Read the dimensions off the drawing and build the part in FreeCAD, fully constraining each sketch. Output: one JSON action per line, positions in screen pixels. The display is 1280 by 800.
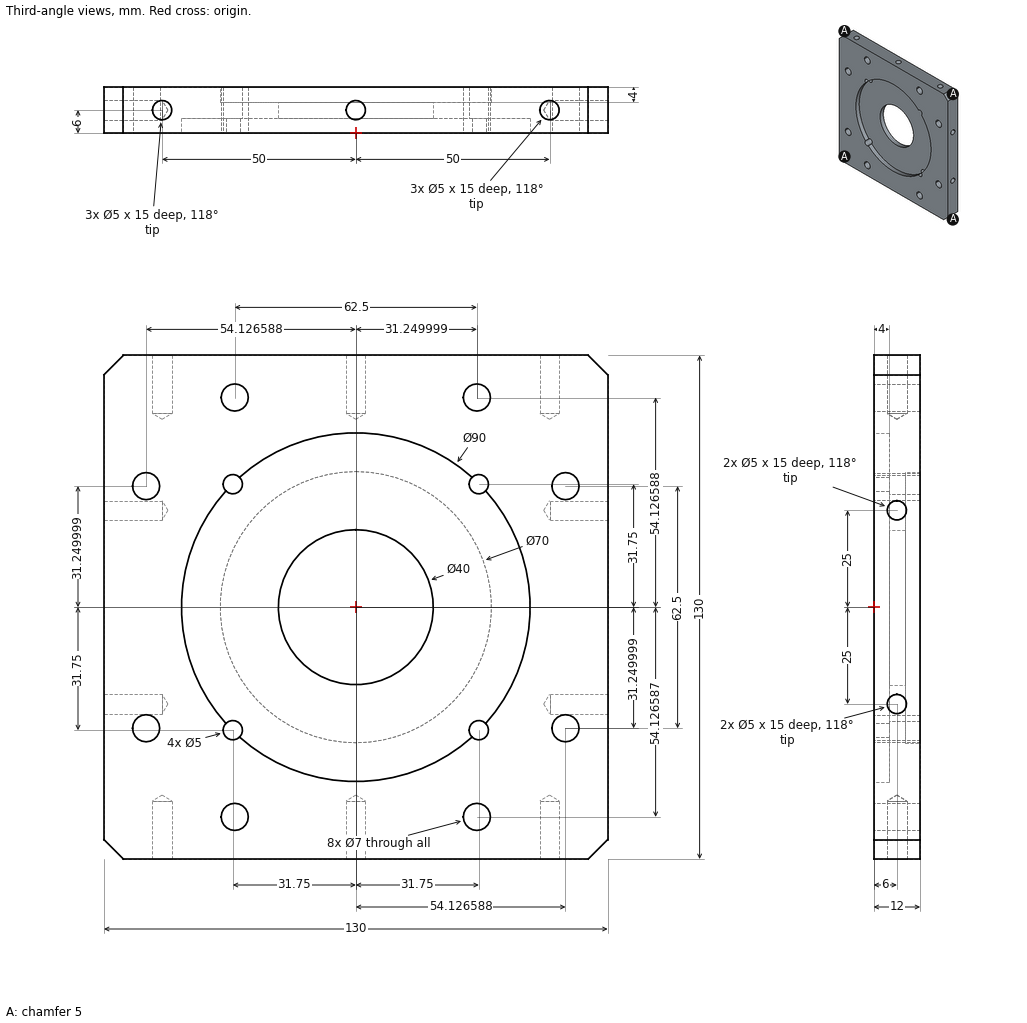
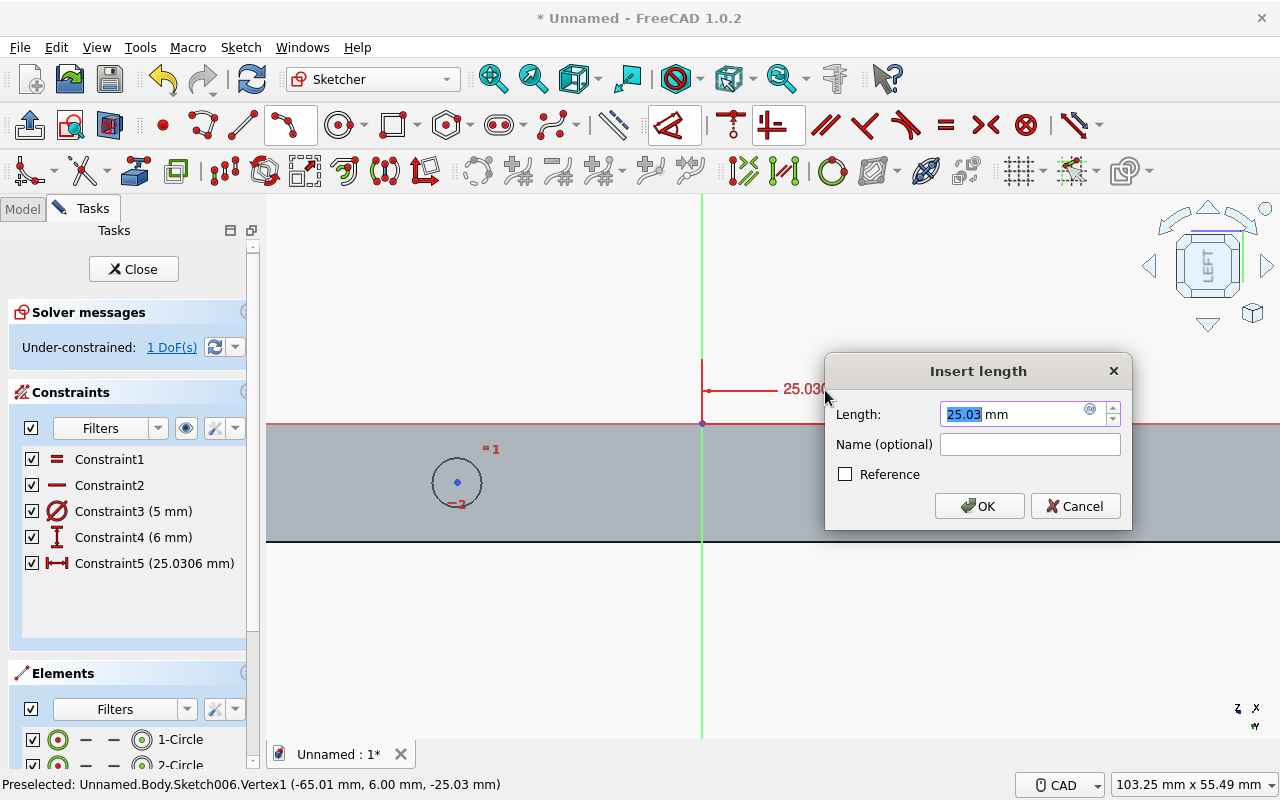
{"action": "type", "text": "25"}
{"action": "key", "text": "Return"}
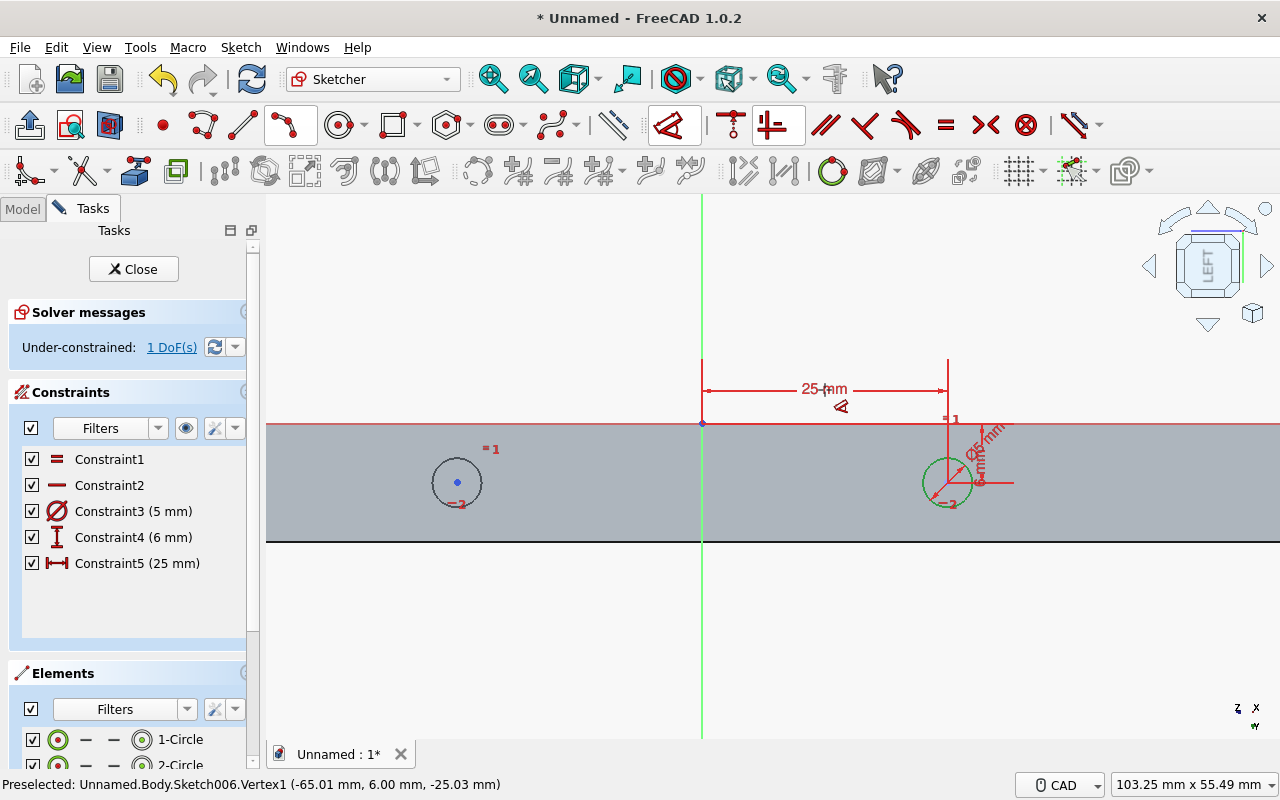
{"action": "left_click", "coordinate": [457, 483]}
{"action": "left_click", "coordinate": [580, 390]}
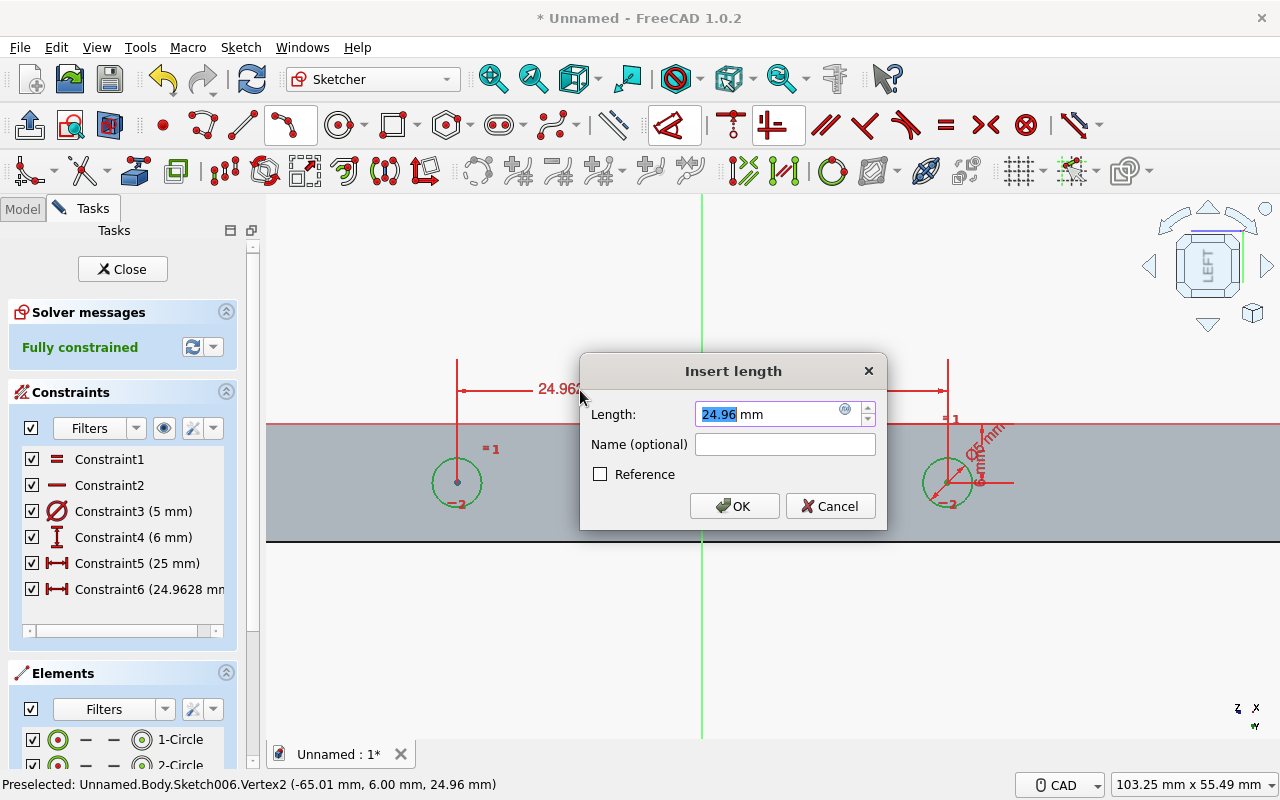
{"action": "type", "text": "25"}
{"action": "key", "text": "Return"}
{"action": "key", "text": "Escape"}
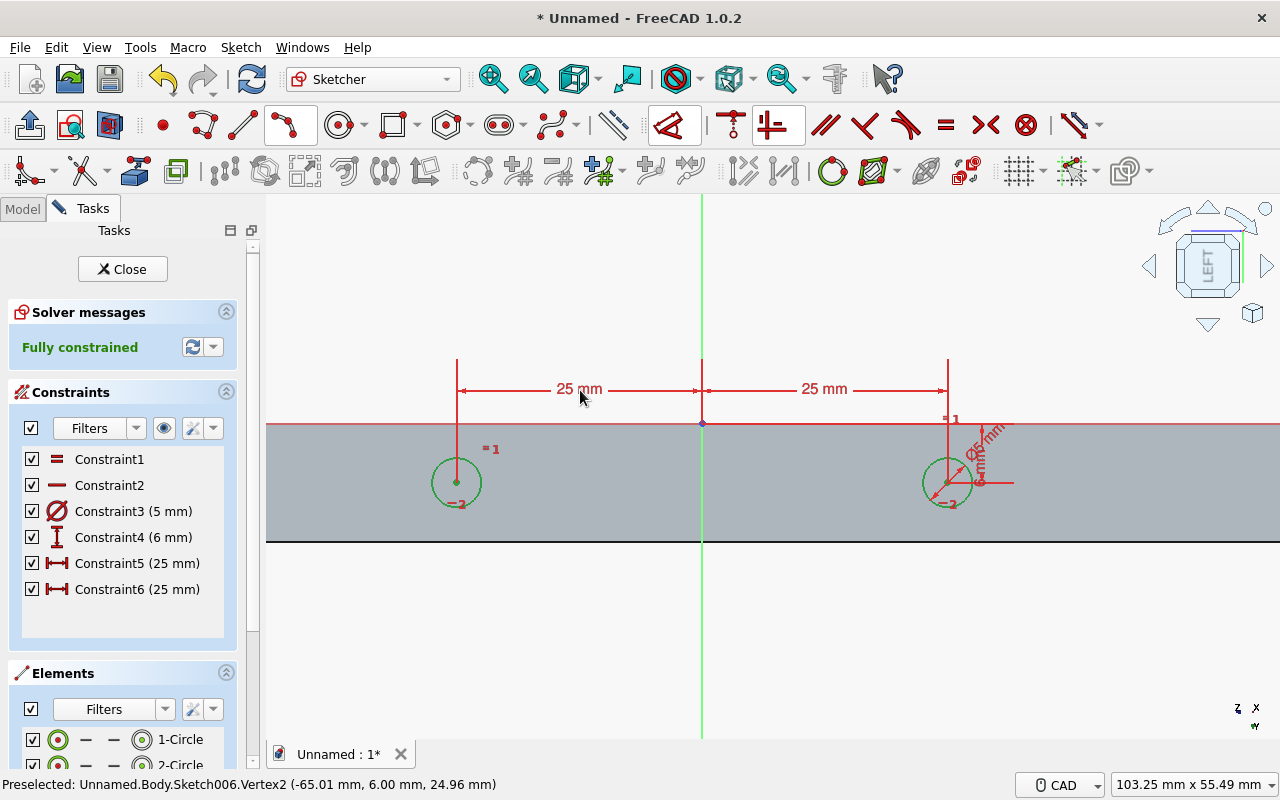
{"action": "left_click", "coordinate": [123, 269]}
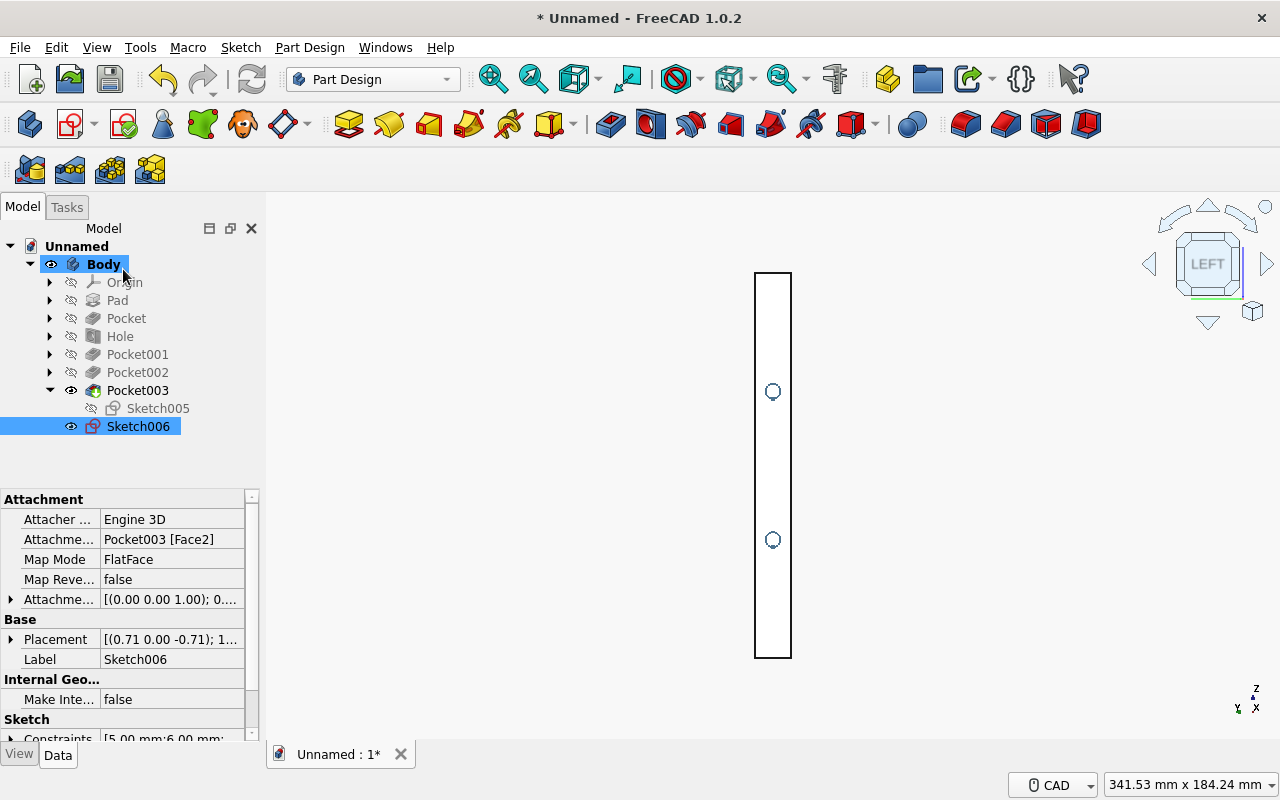
{"action": "left_click", "coordinate": [652, 124]}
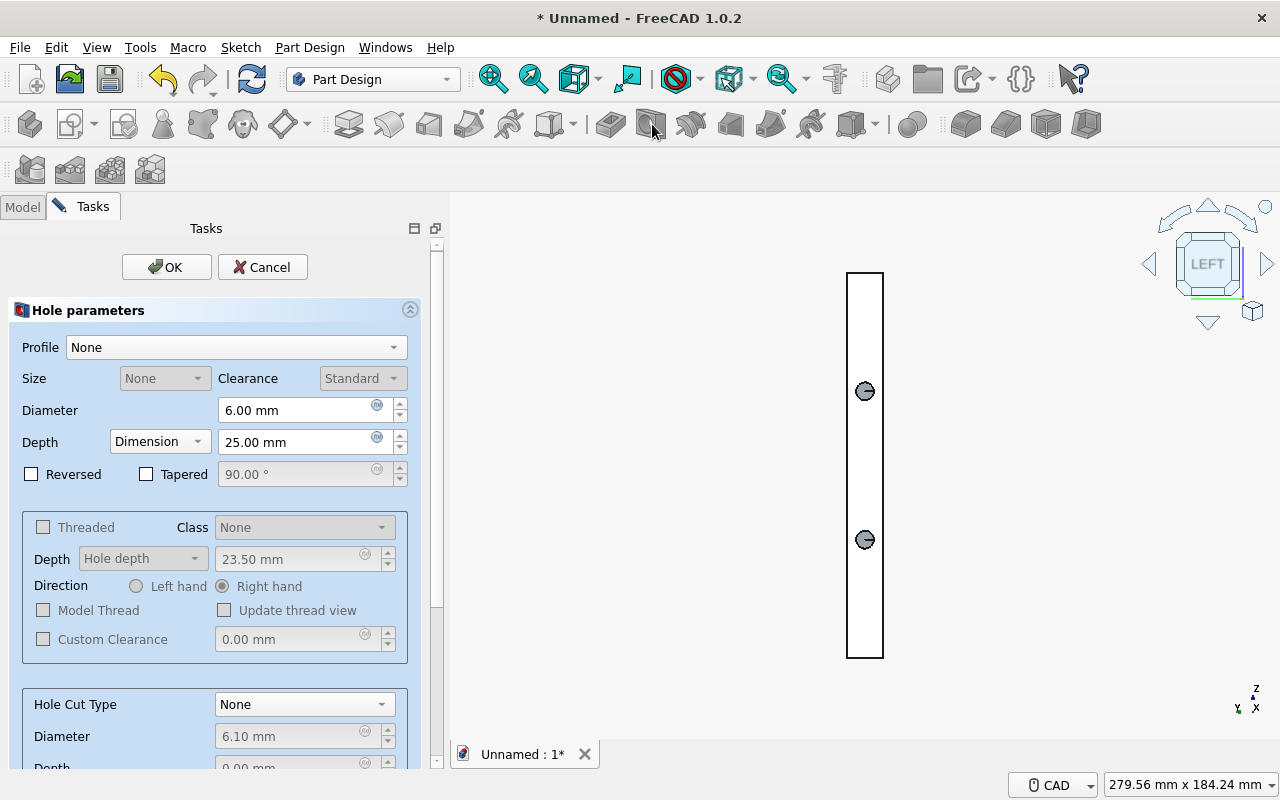
{"action": "triple_click", "coordinate": [305, 410]}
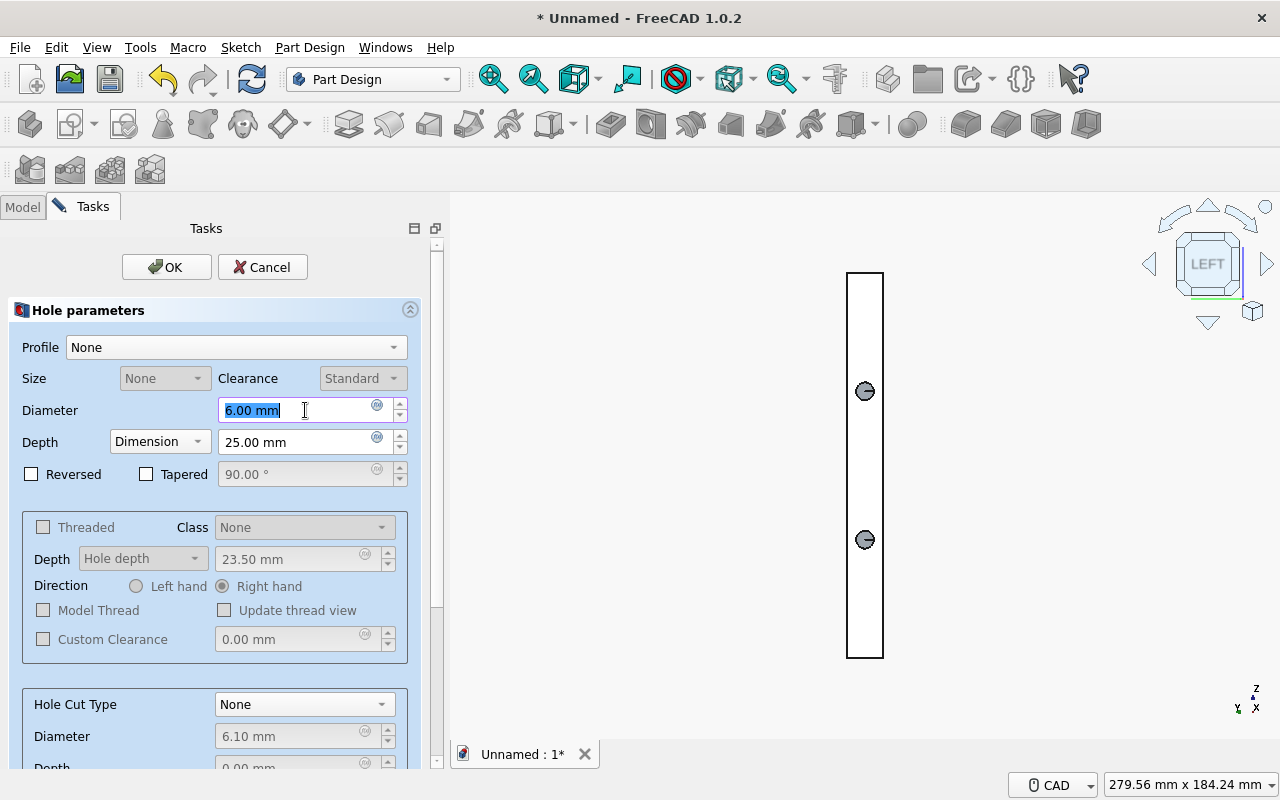
{"action": "type", "text": "5"}
{"action": "key", "text": "Tab"}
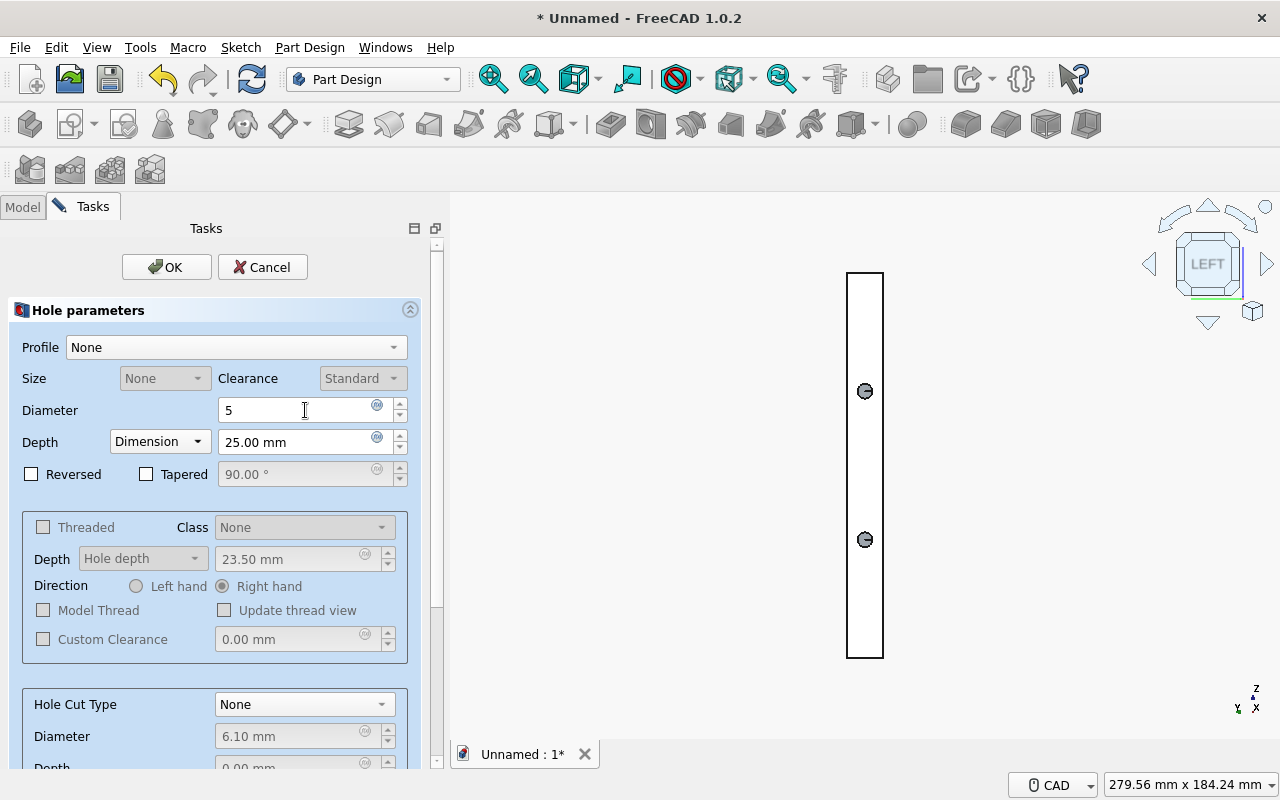
{"action": "triple_click", "coordinate": [305, 442]}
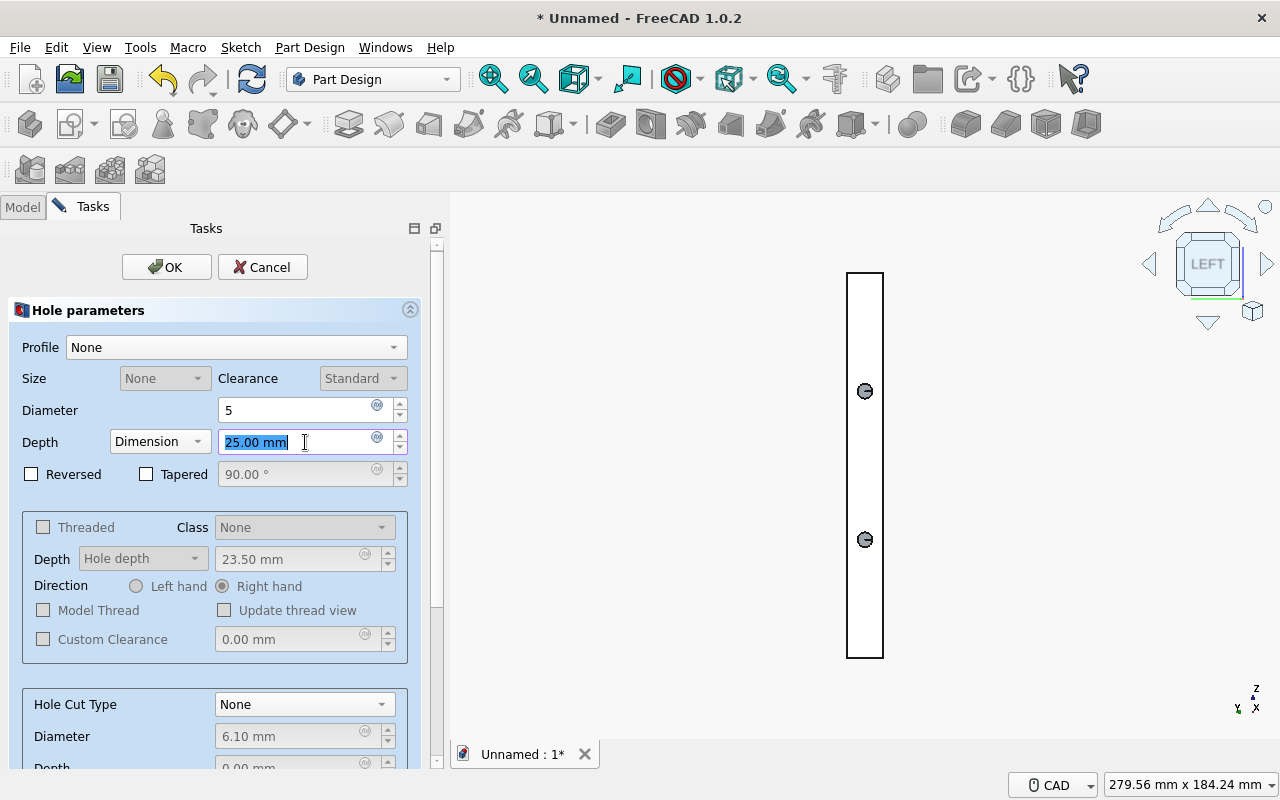
{"action": "type", "text": "15"}
{"action": "key", "text": "Tab"}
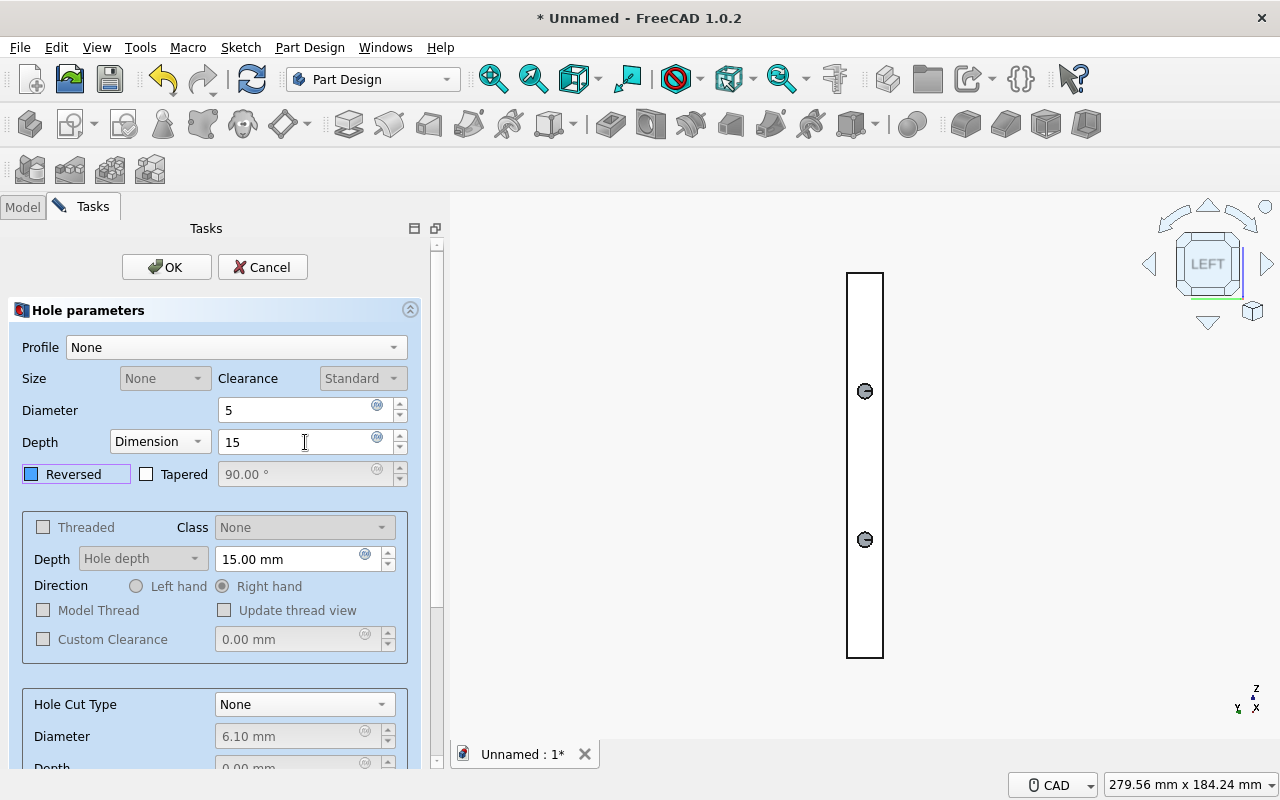
{"action": "left_click", "coordinate": [167, 267]}